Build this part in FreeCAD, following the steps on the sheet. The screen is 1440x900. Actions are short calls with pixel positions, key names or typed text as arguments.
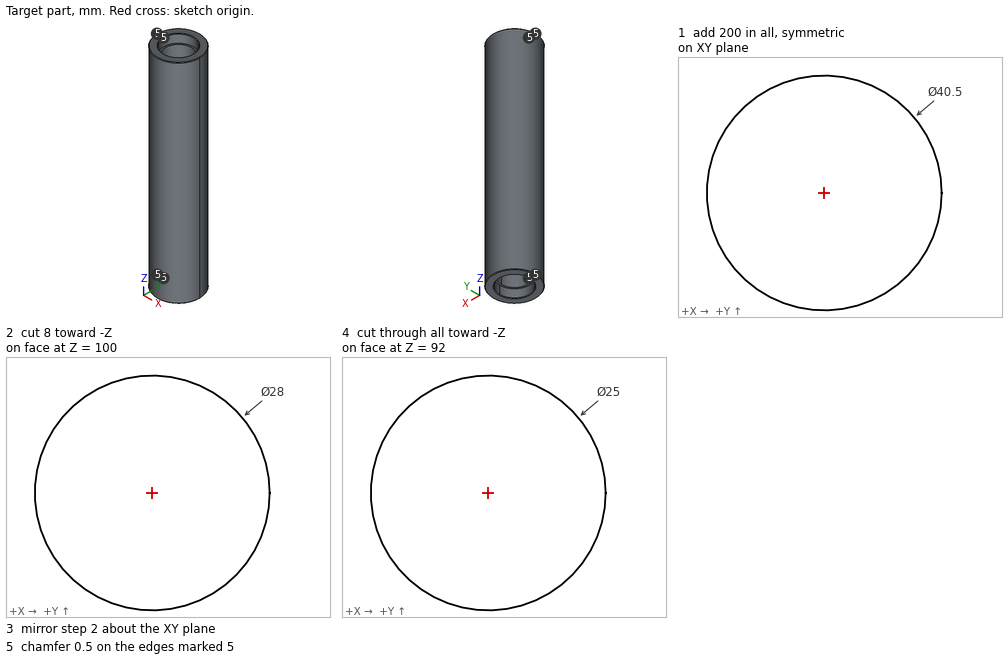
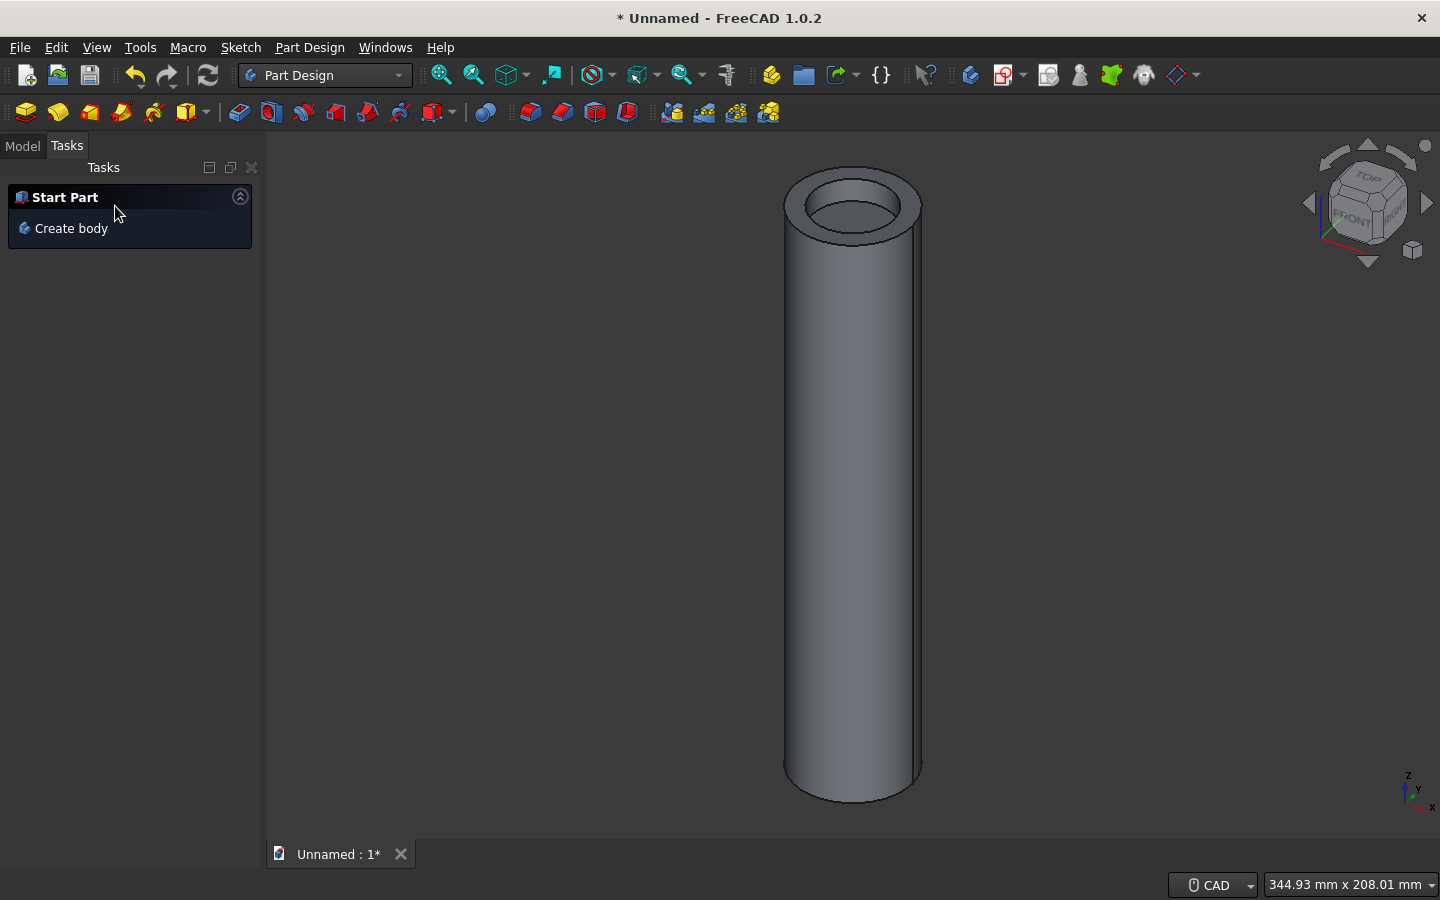
click(23, 145)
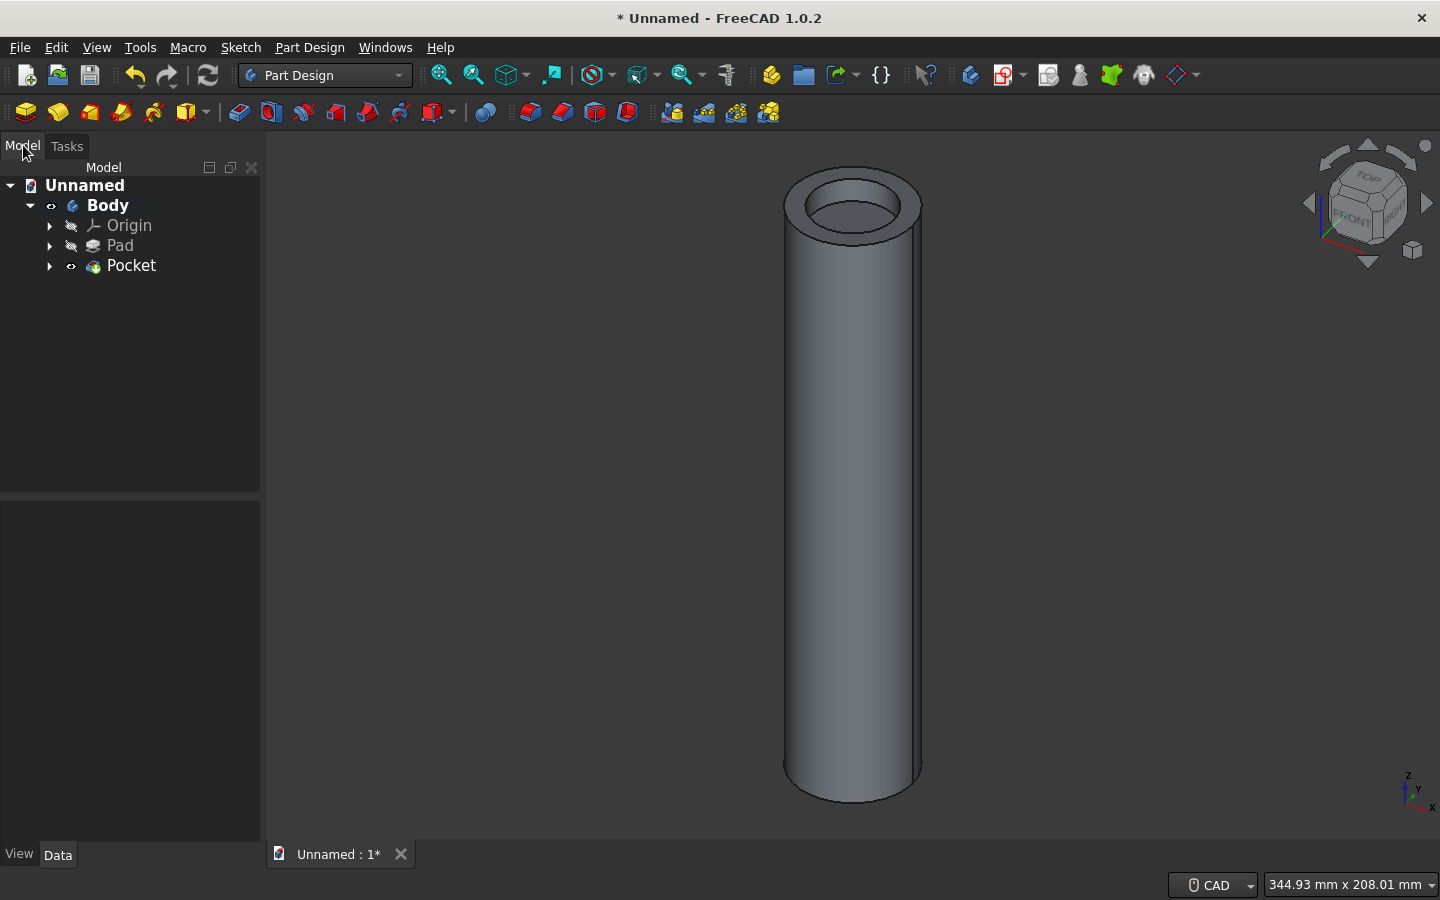
click(116, 266)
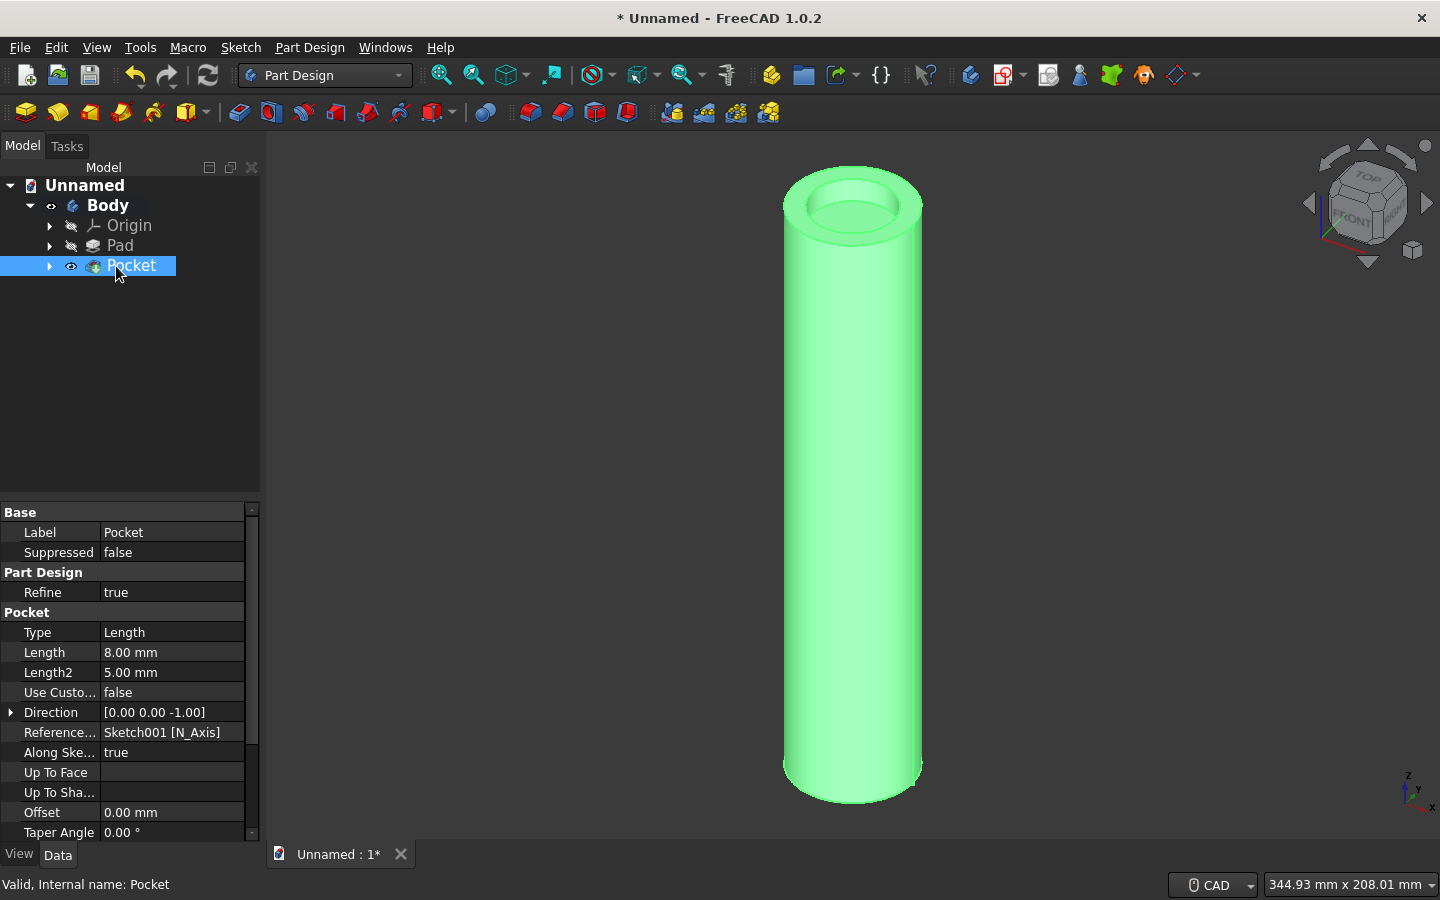
click(672, 112)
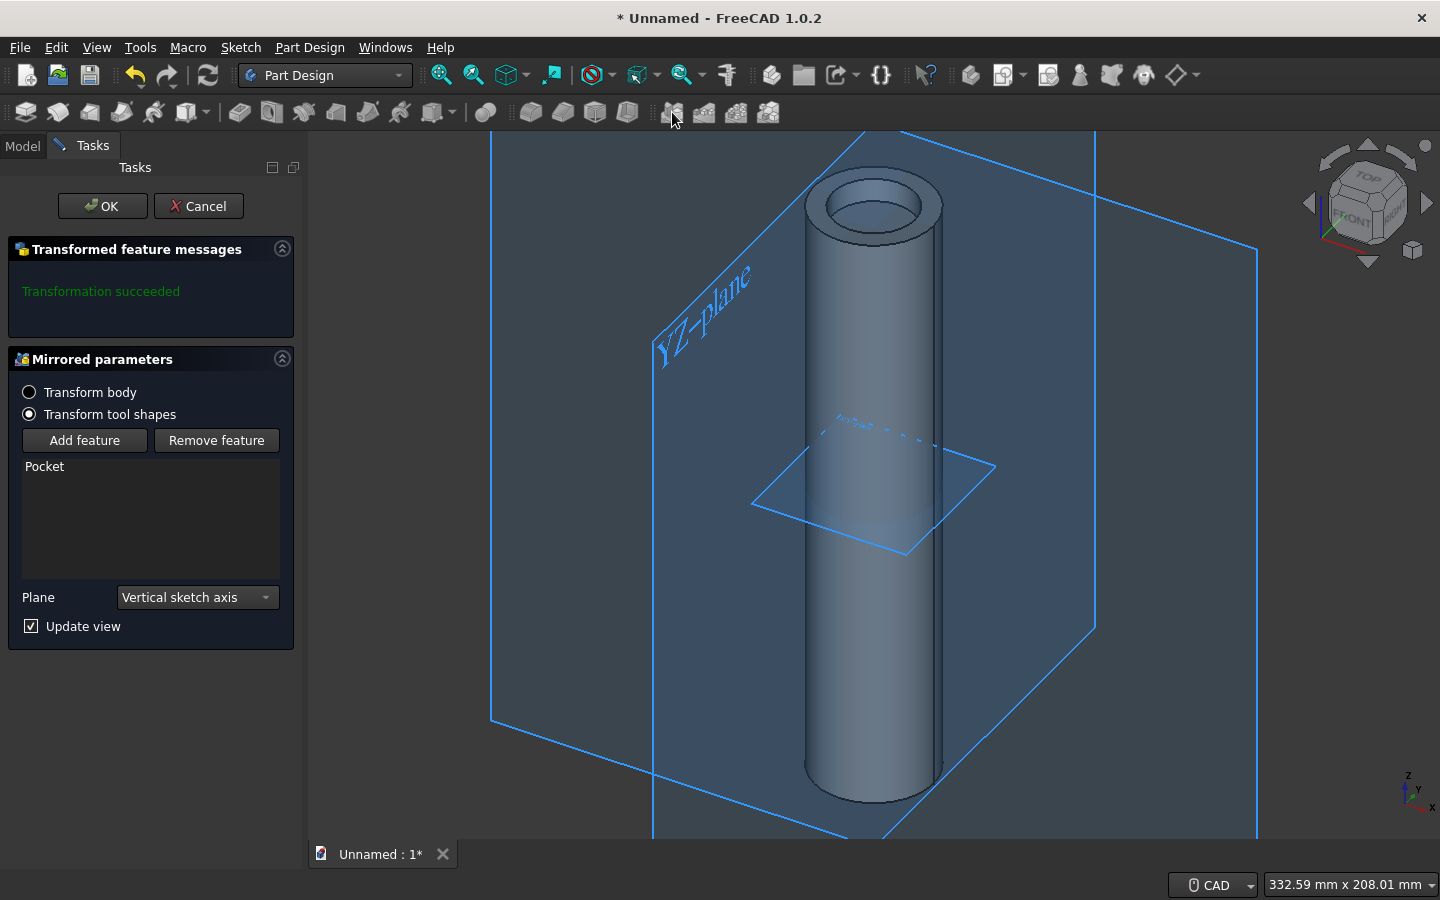
click(198, 598)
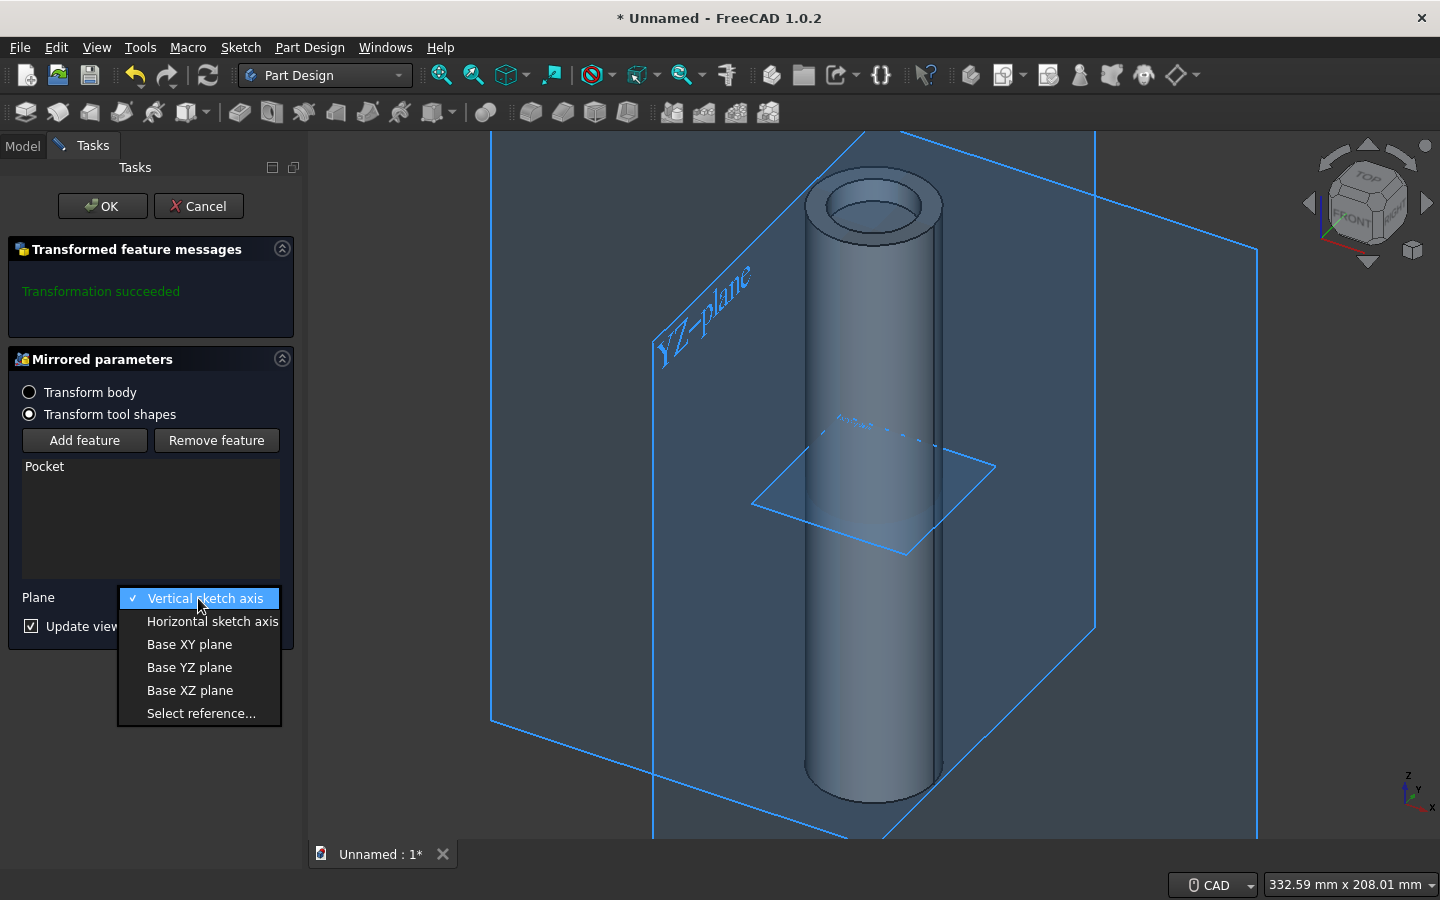
click(198, 644)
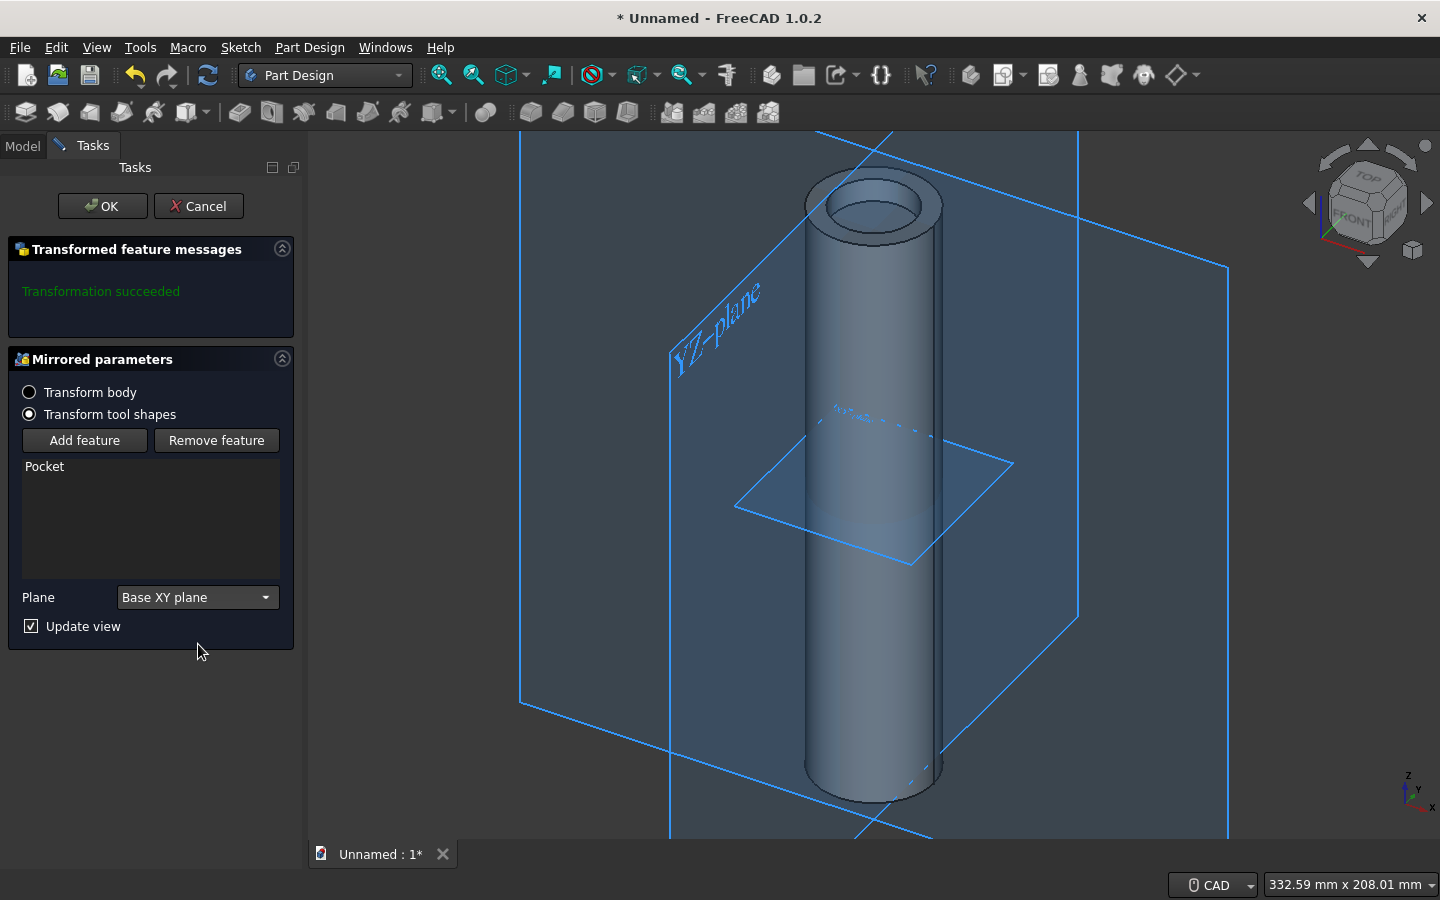
click(103, 206)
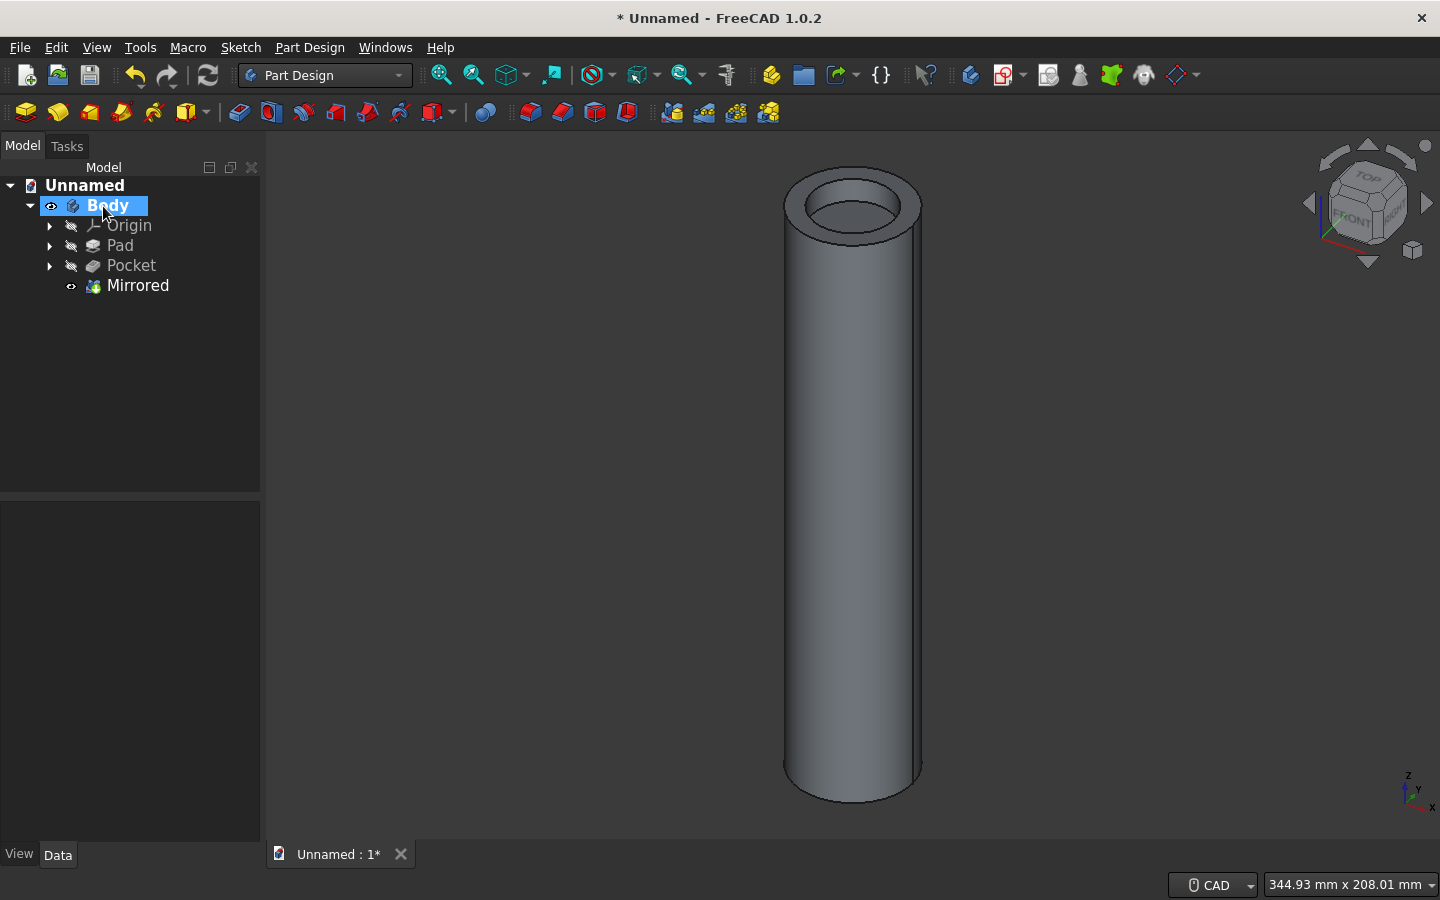
click(860, 221)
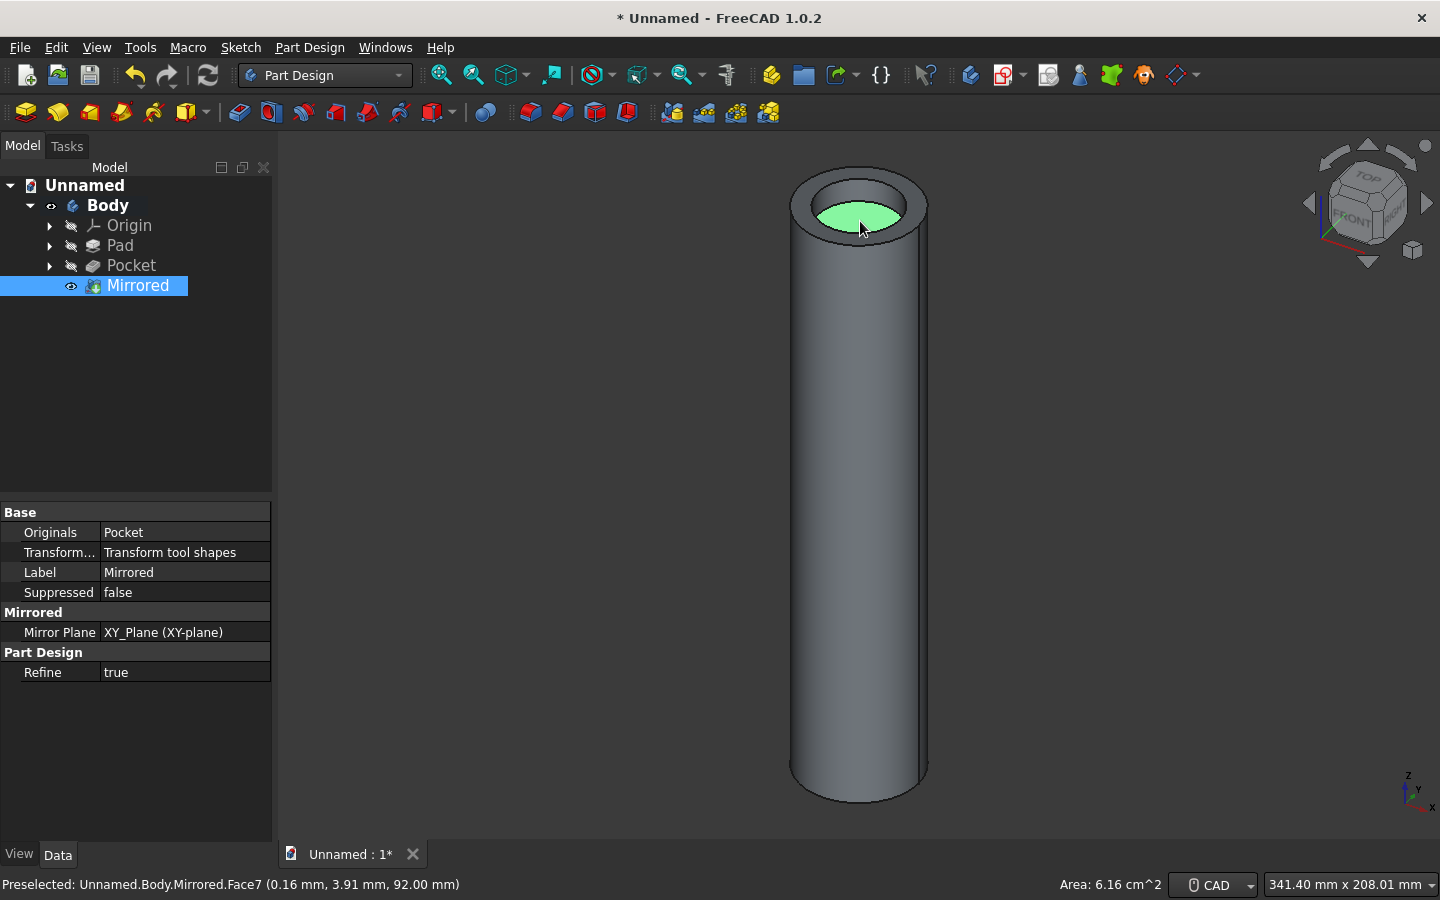
click(1004, 76)